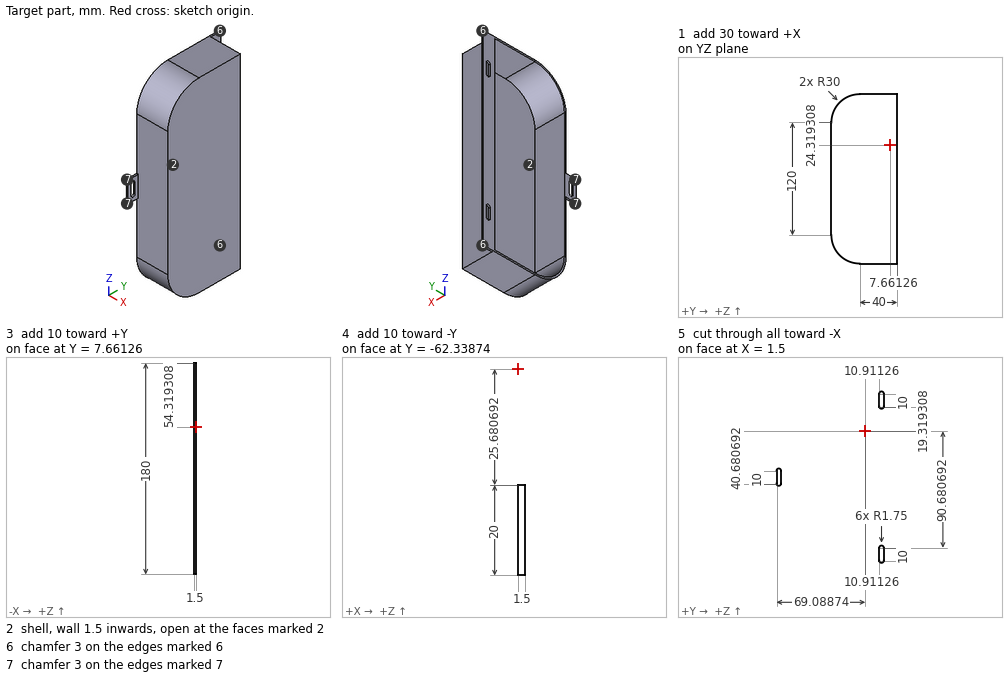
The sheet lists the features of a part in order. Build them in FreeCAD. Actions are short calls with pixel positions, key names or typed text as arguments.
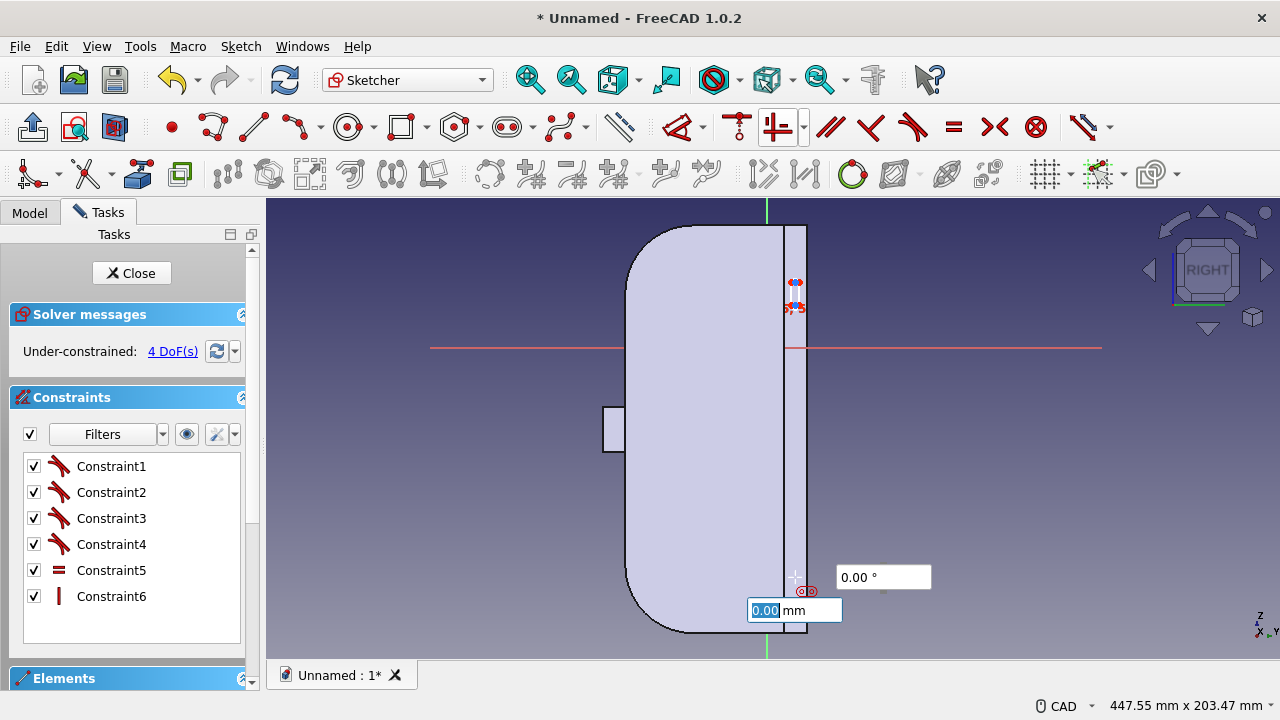
click(795, 554)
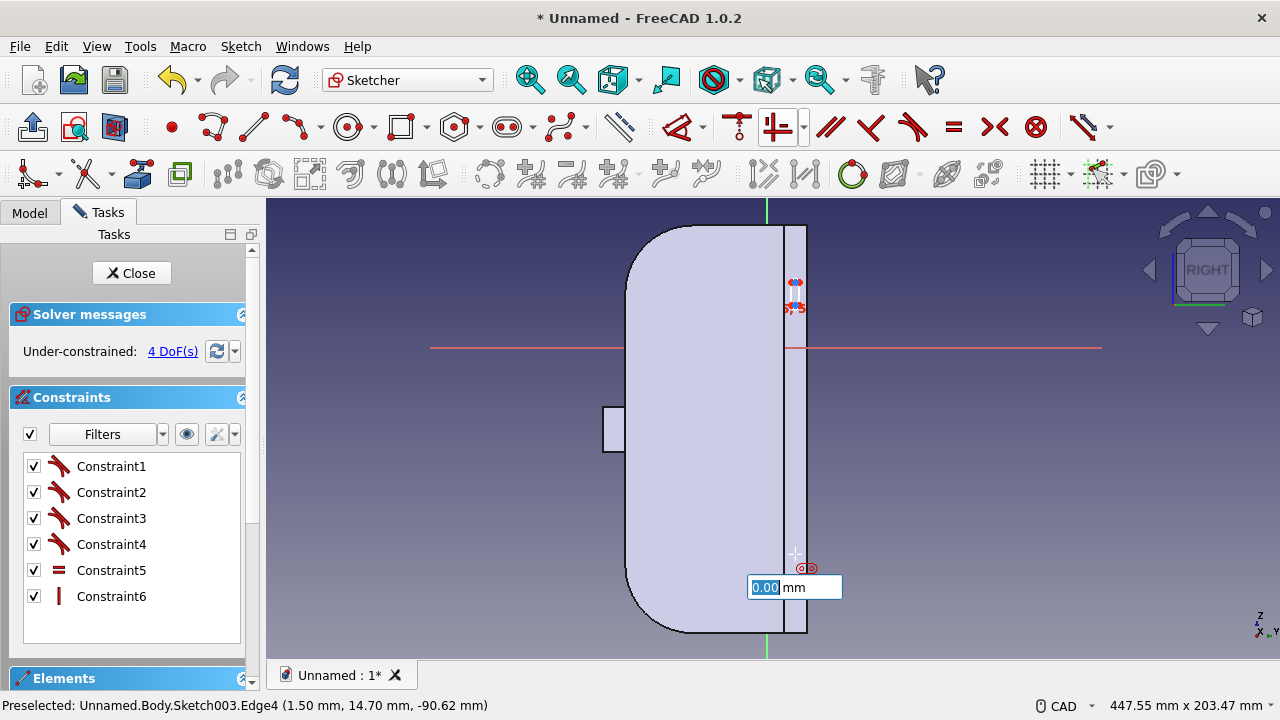
scroll(799, 565, up, 7)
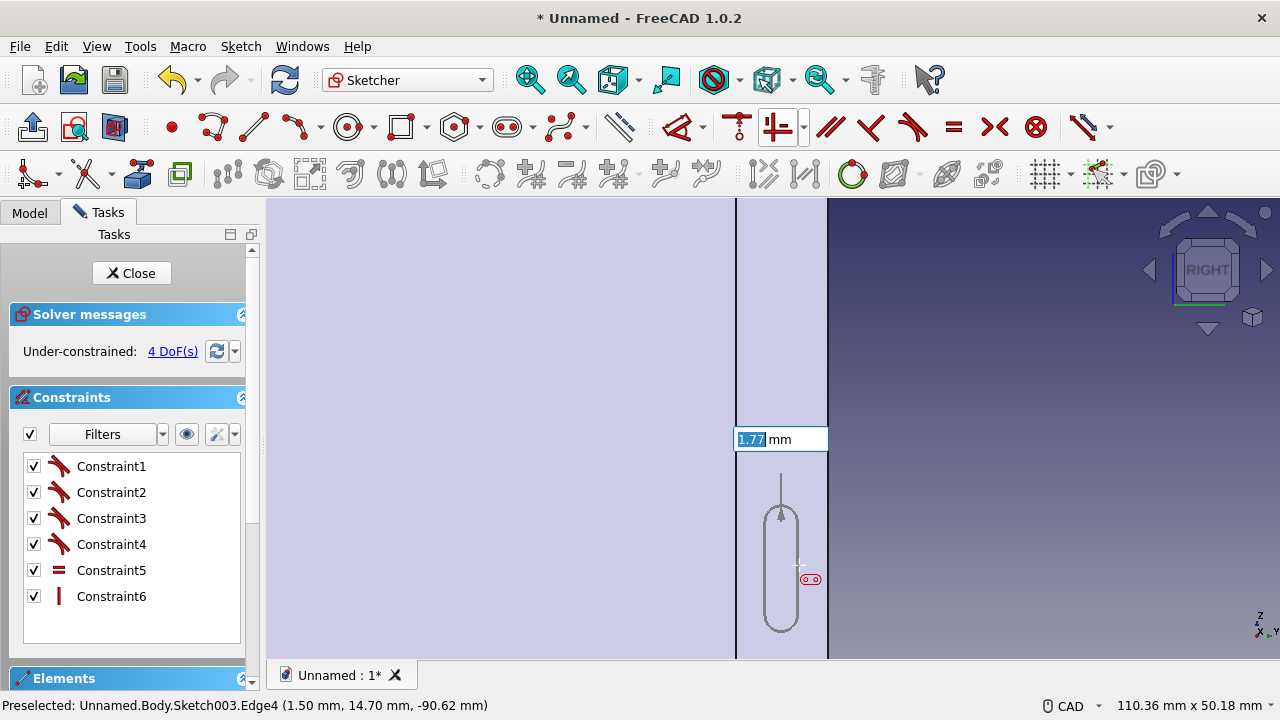
click(798, 564)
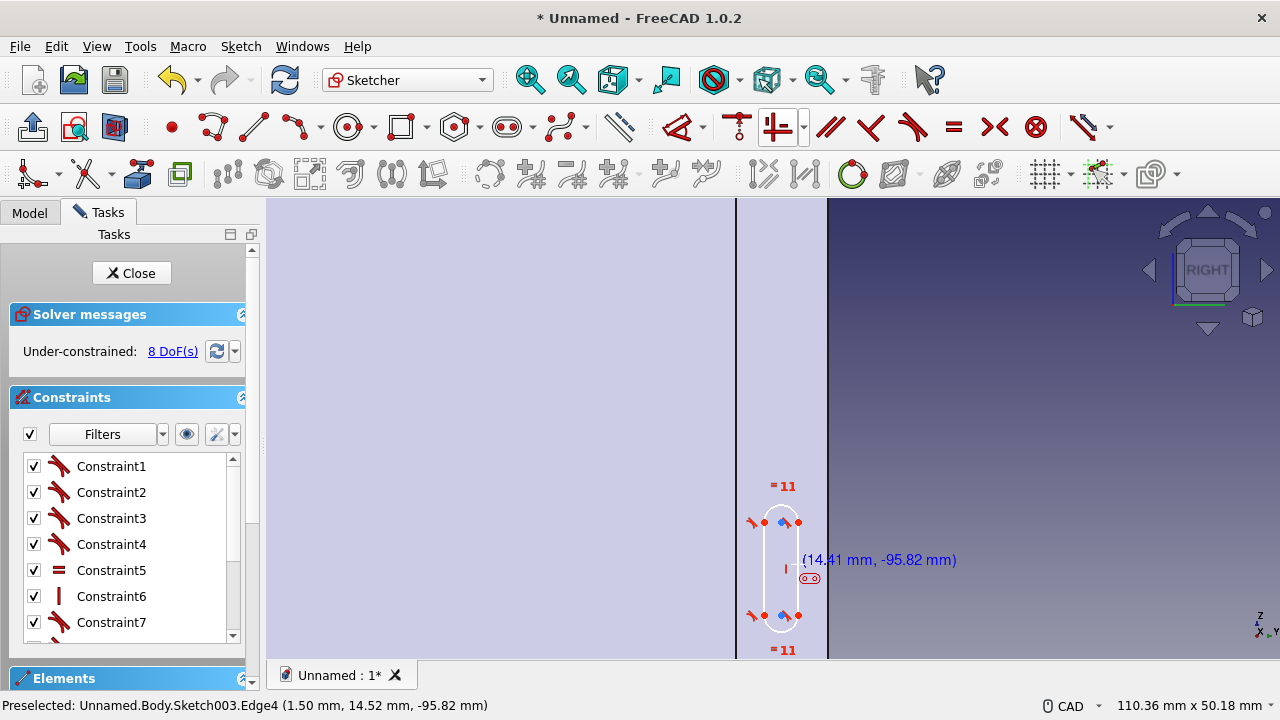
scroll(799, 565, down, 7)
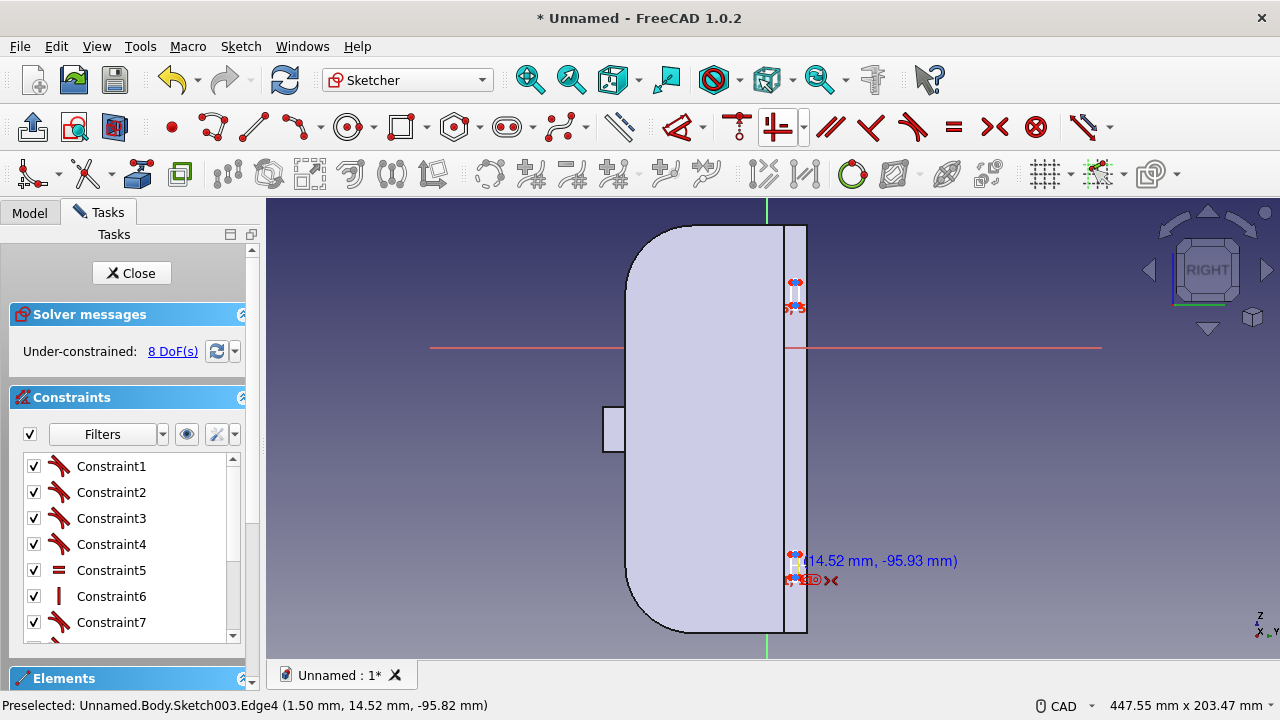
scroll(614, 441, up, 9)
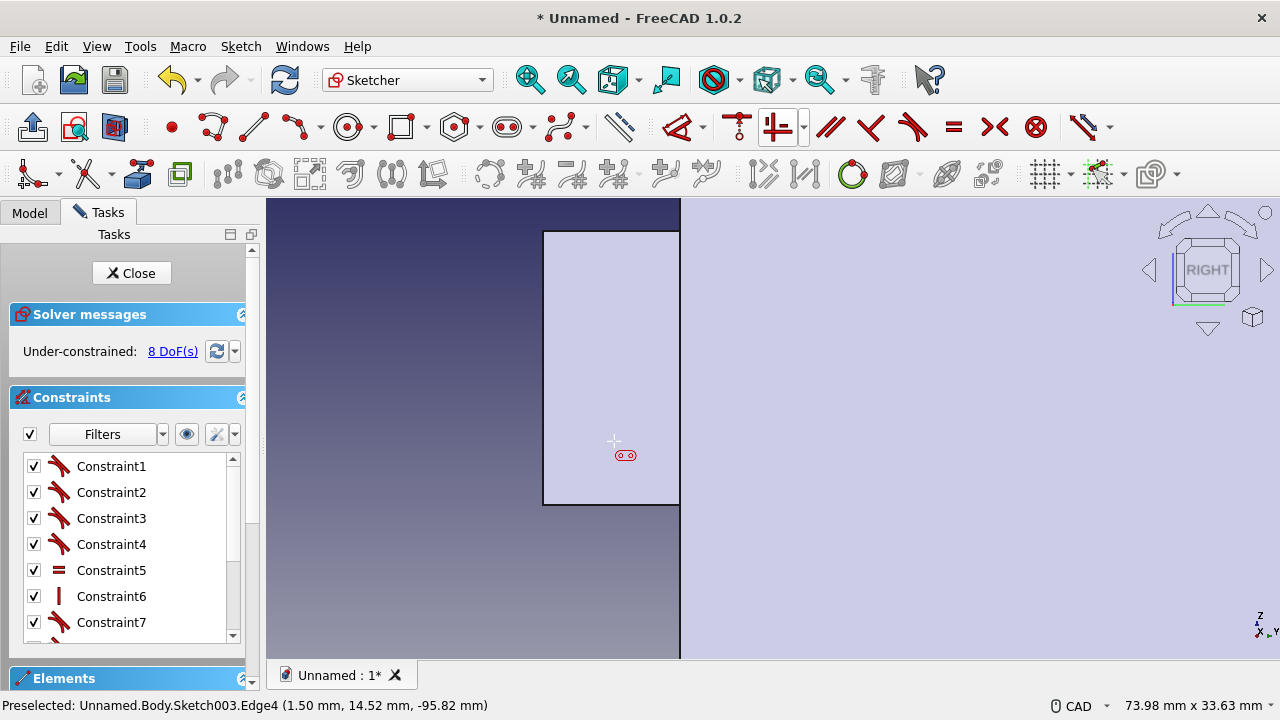
scroll(614, 441, down, 9)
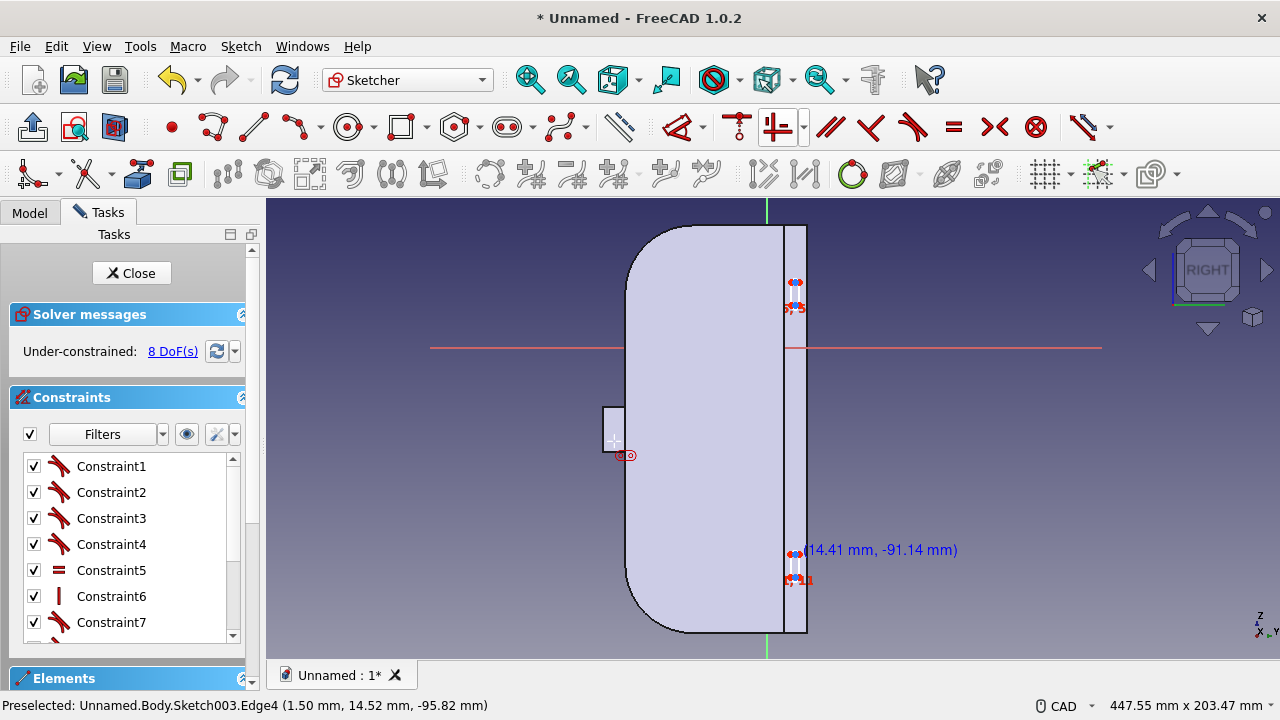
click(614, 441)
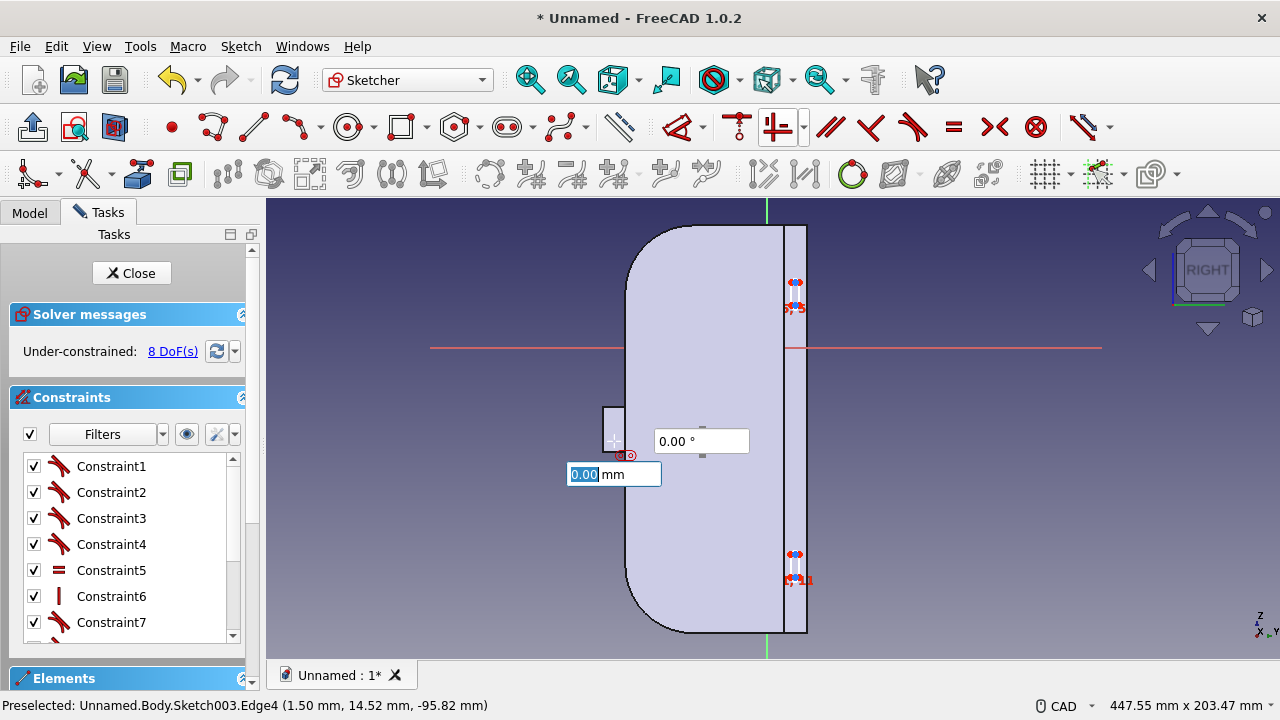
click(614, 418)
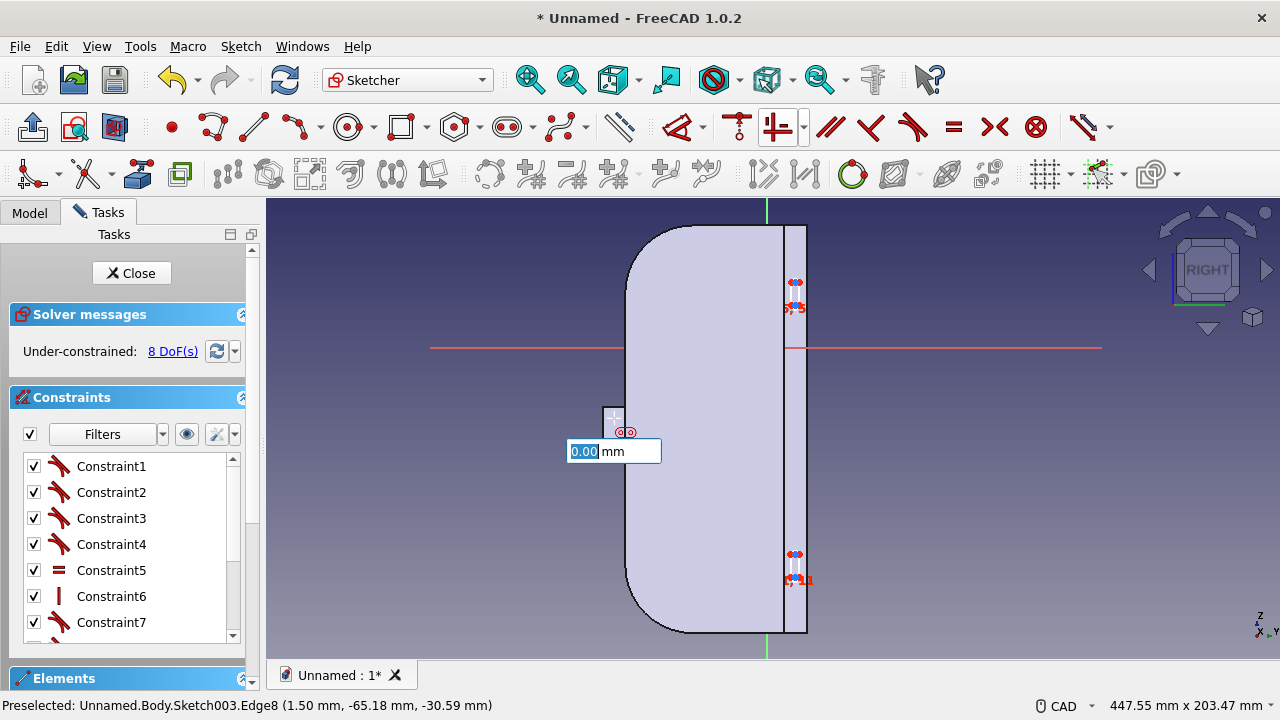
scroll(618, 429, up, 7)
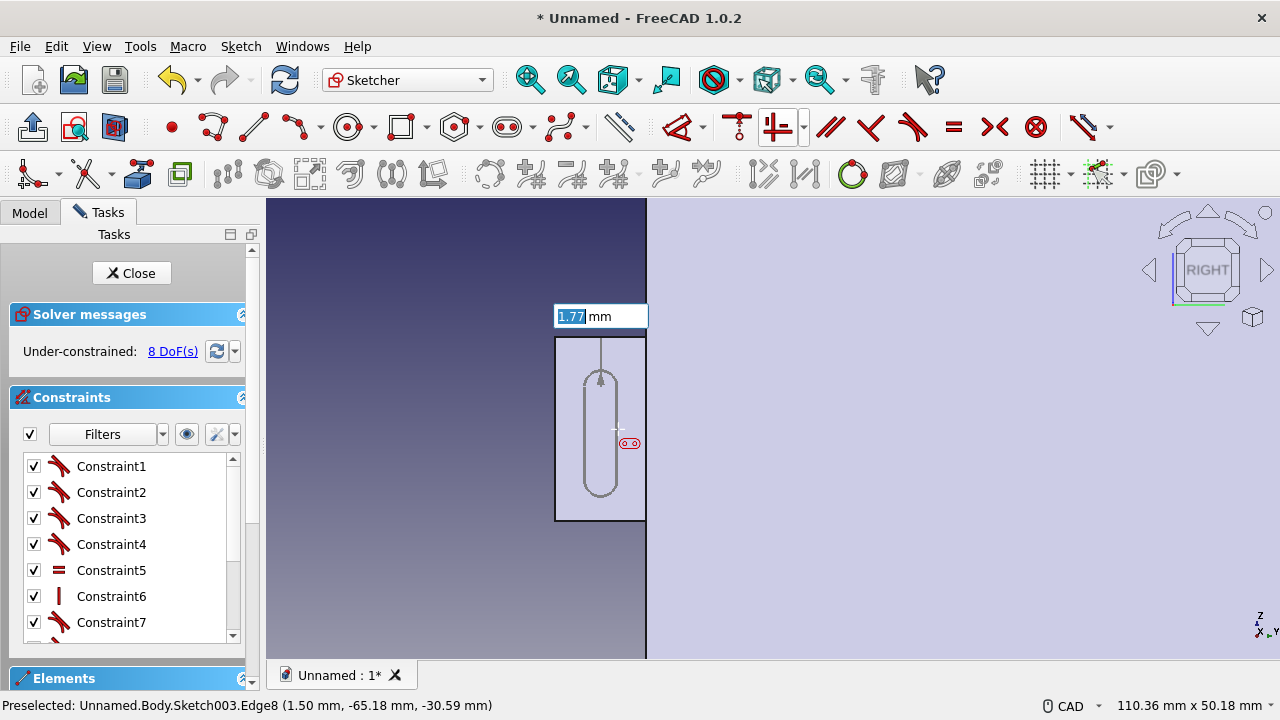
click(617, 429)
key(Escape)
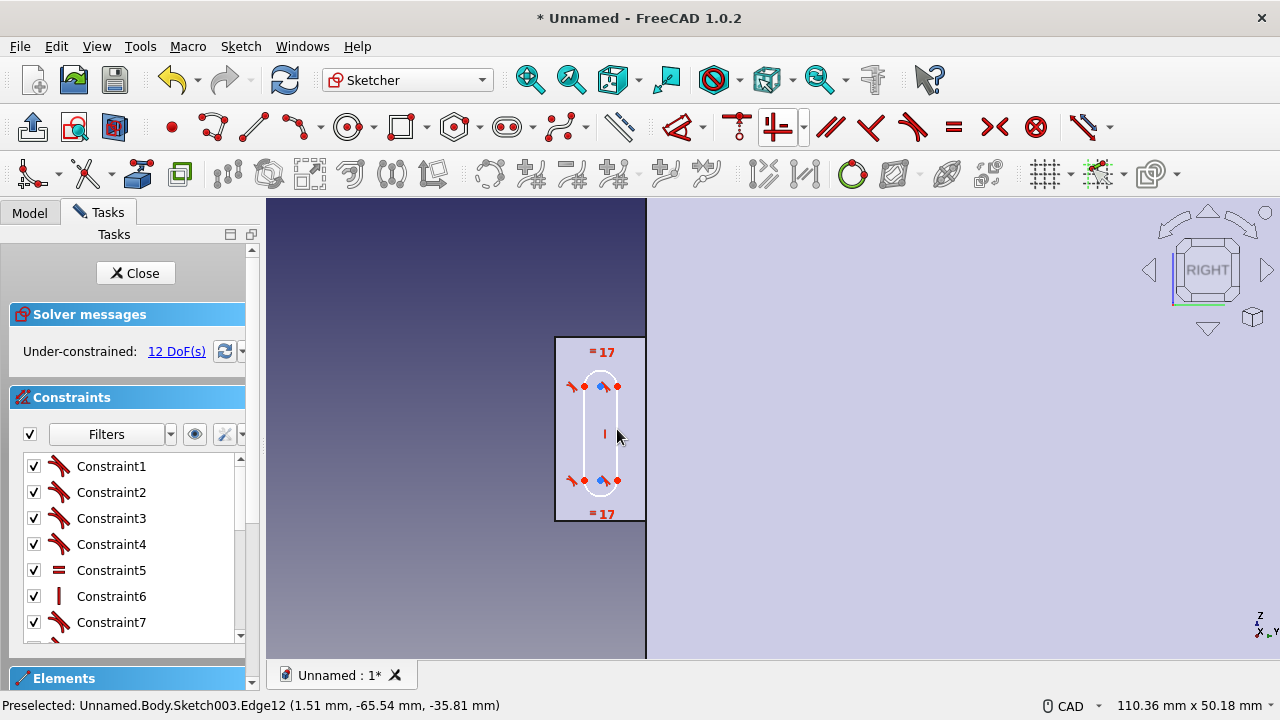
scroll(618, 428, down, 7)